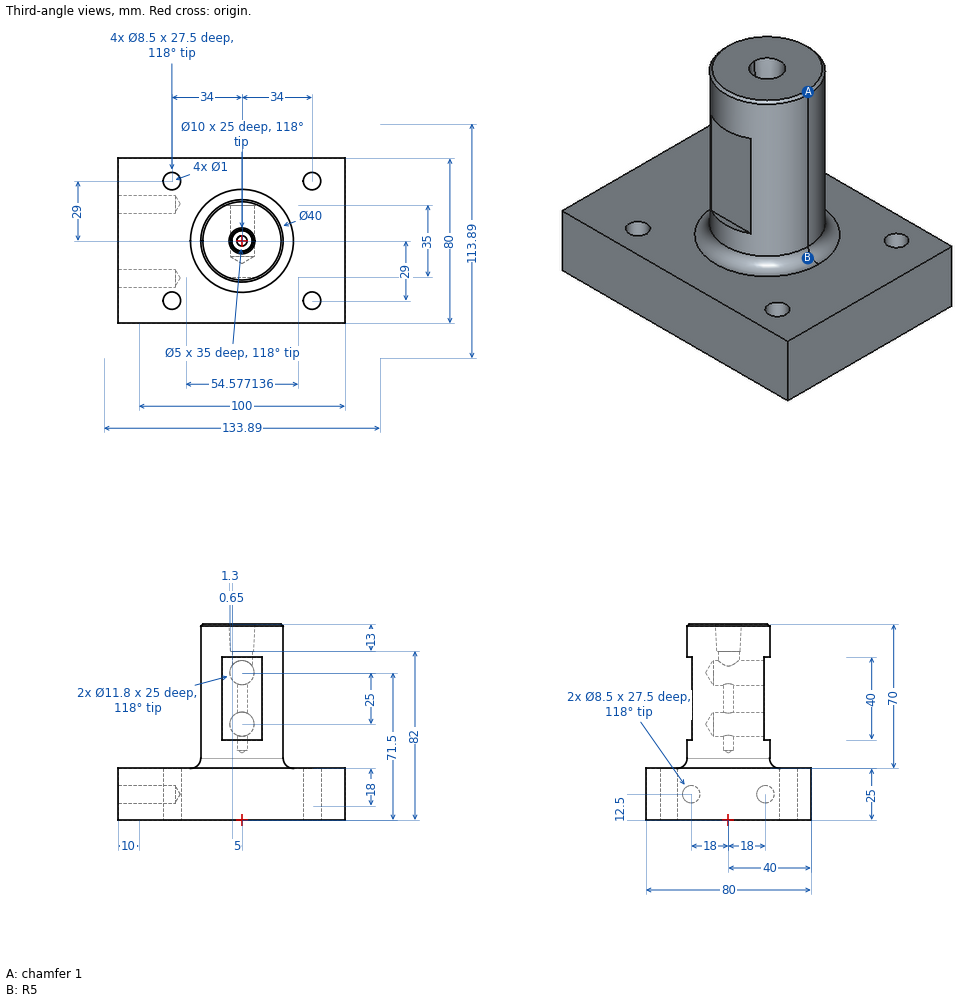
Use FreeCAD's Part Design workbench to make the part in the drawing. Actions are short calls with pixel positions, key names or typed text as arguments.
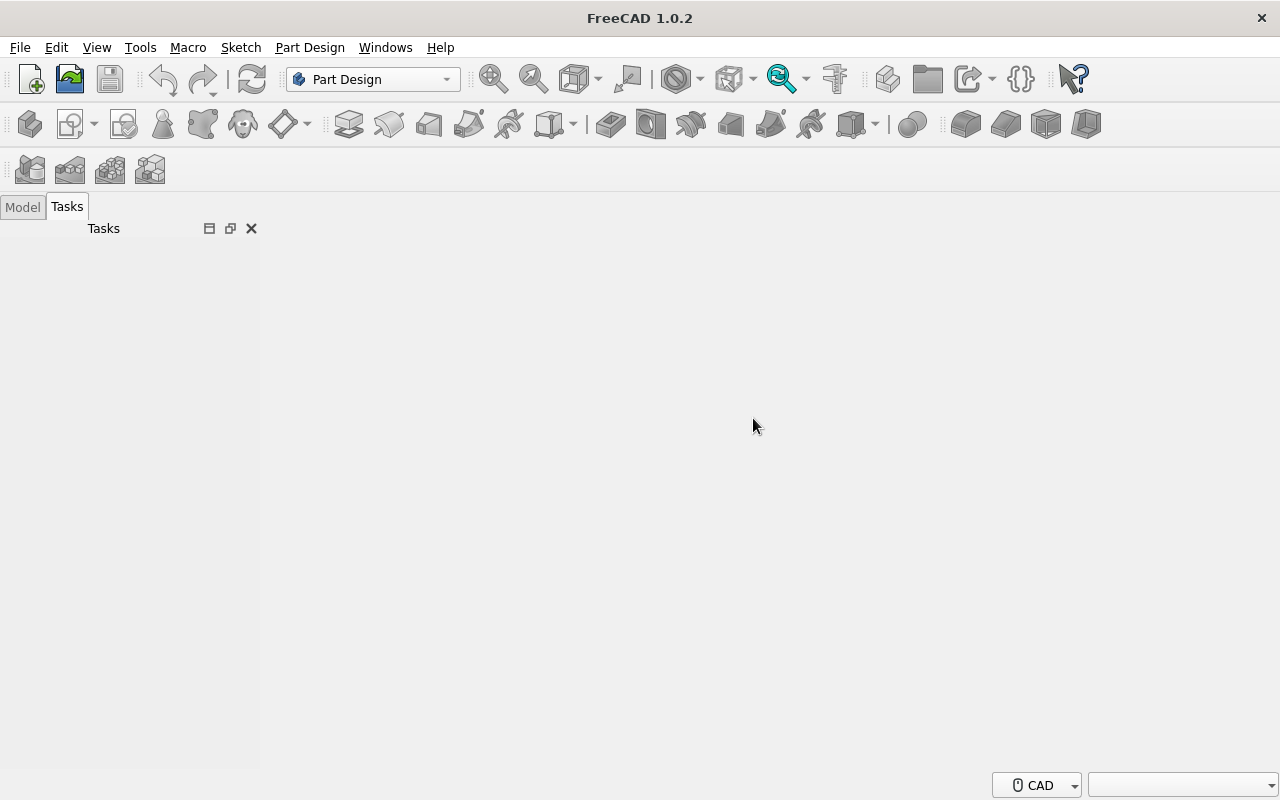
key(ctrl+n)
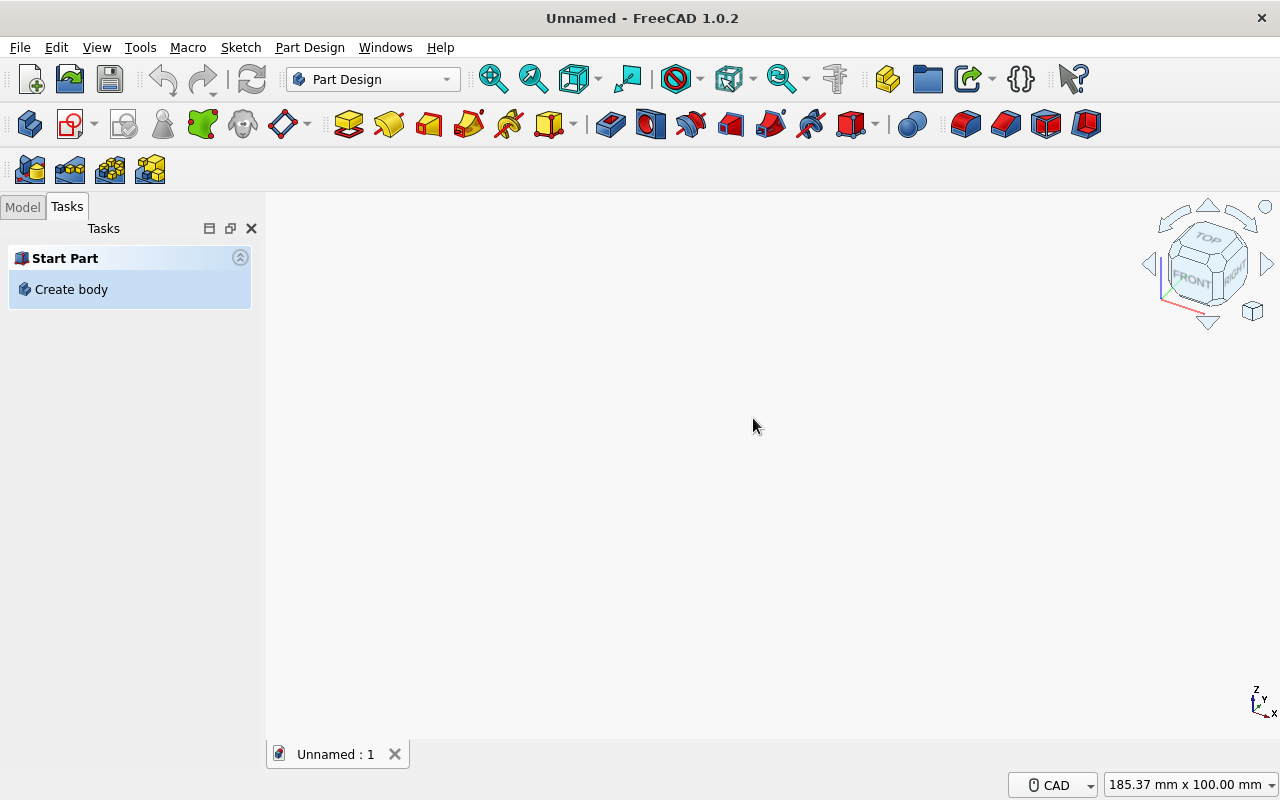
click(70, 124)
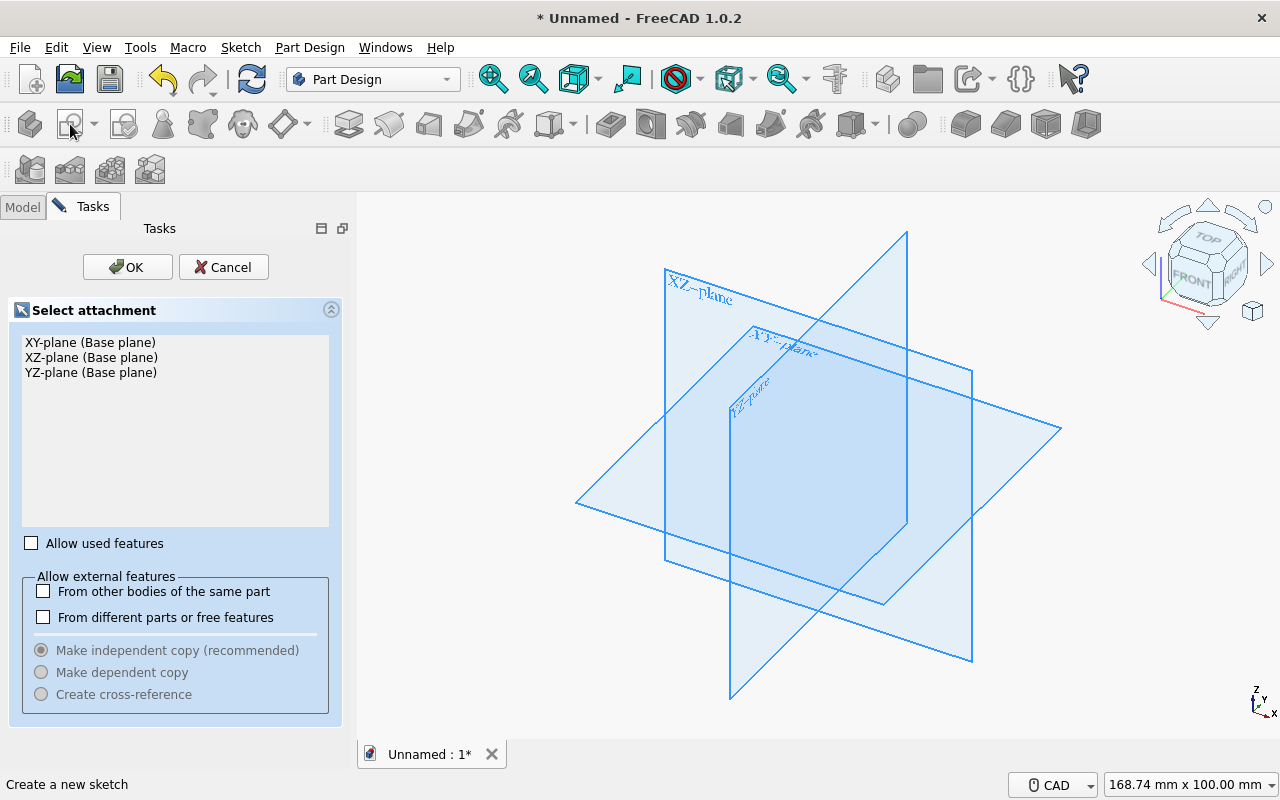
click(82, 342)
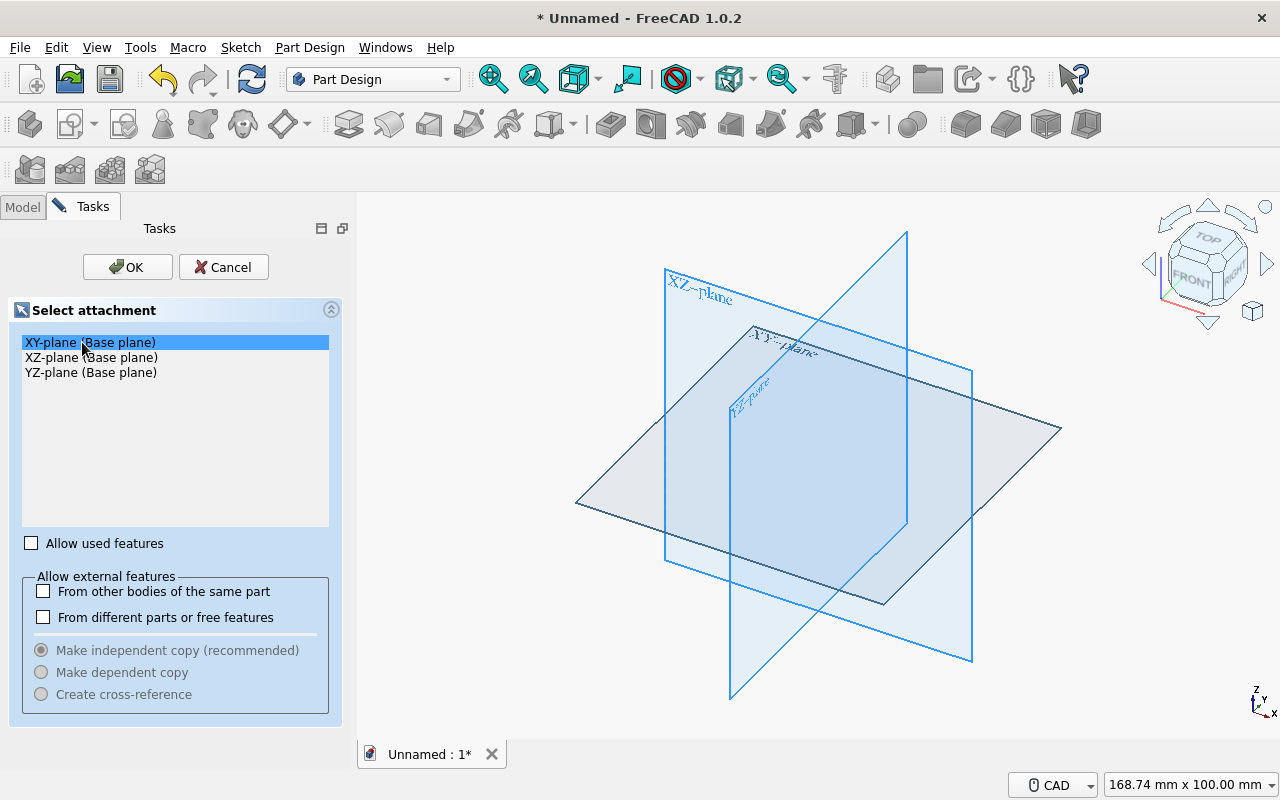
click(128, 267)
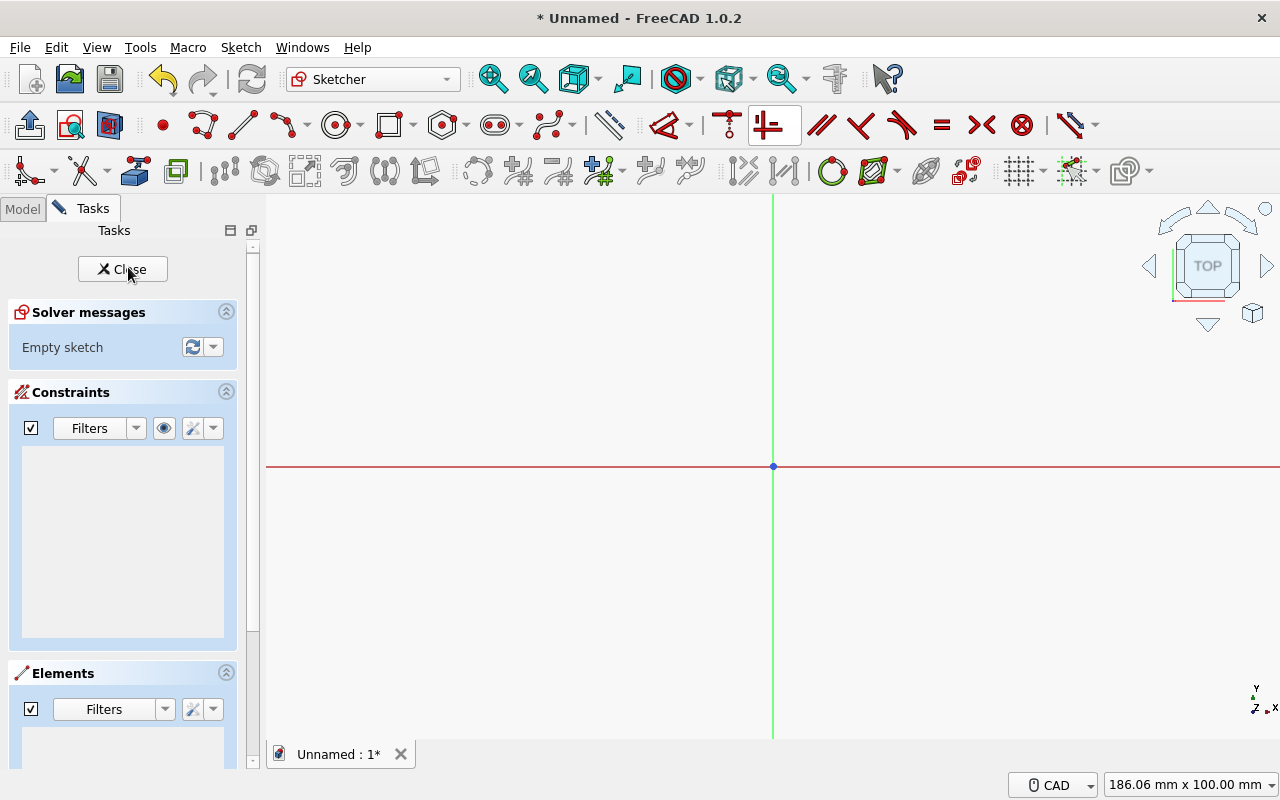
key(g)
key(v)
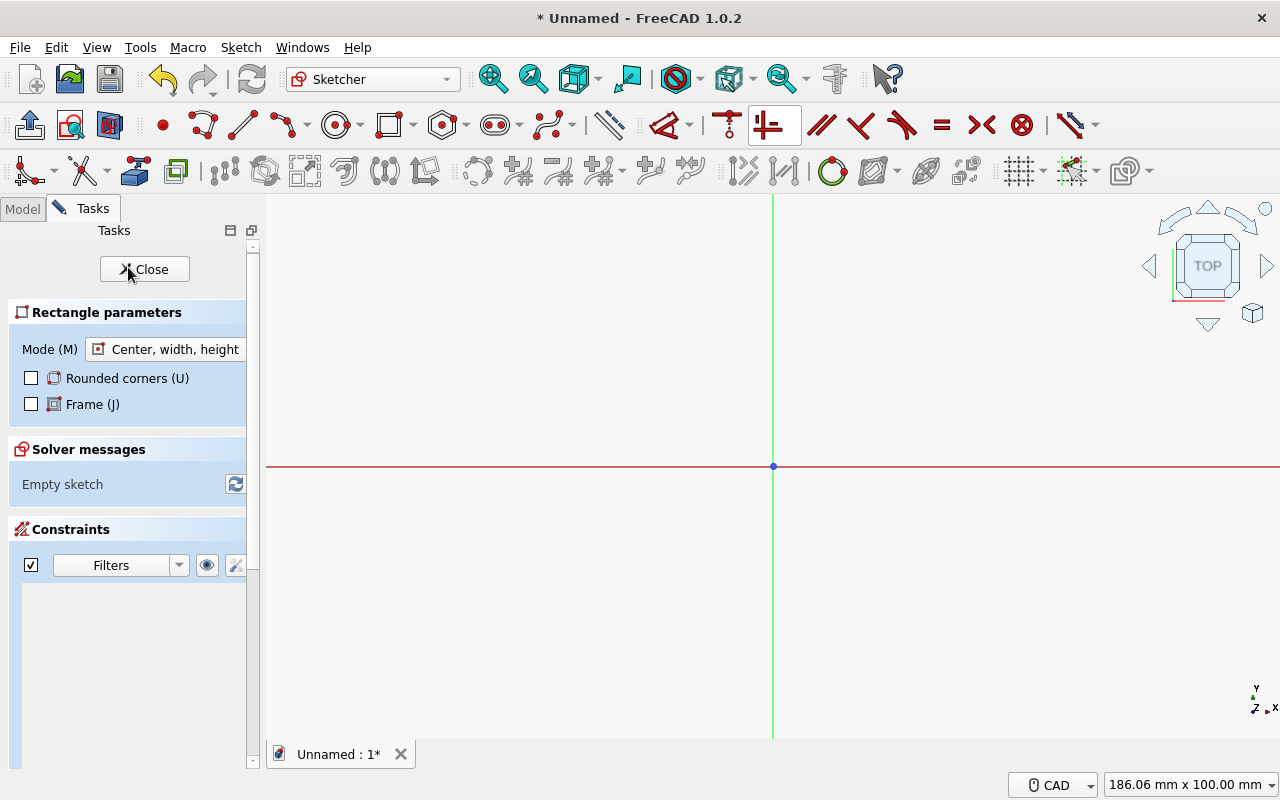
click(773, 466)
click(1046, 248)
key(Escape)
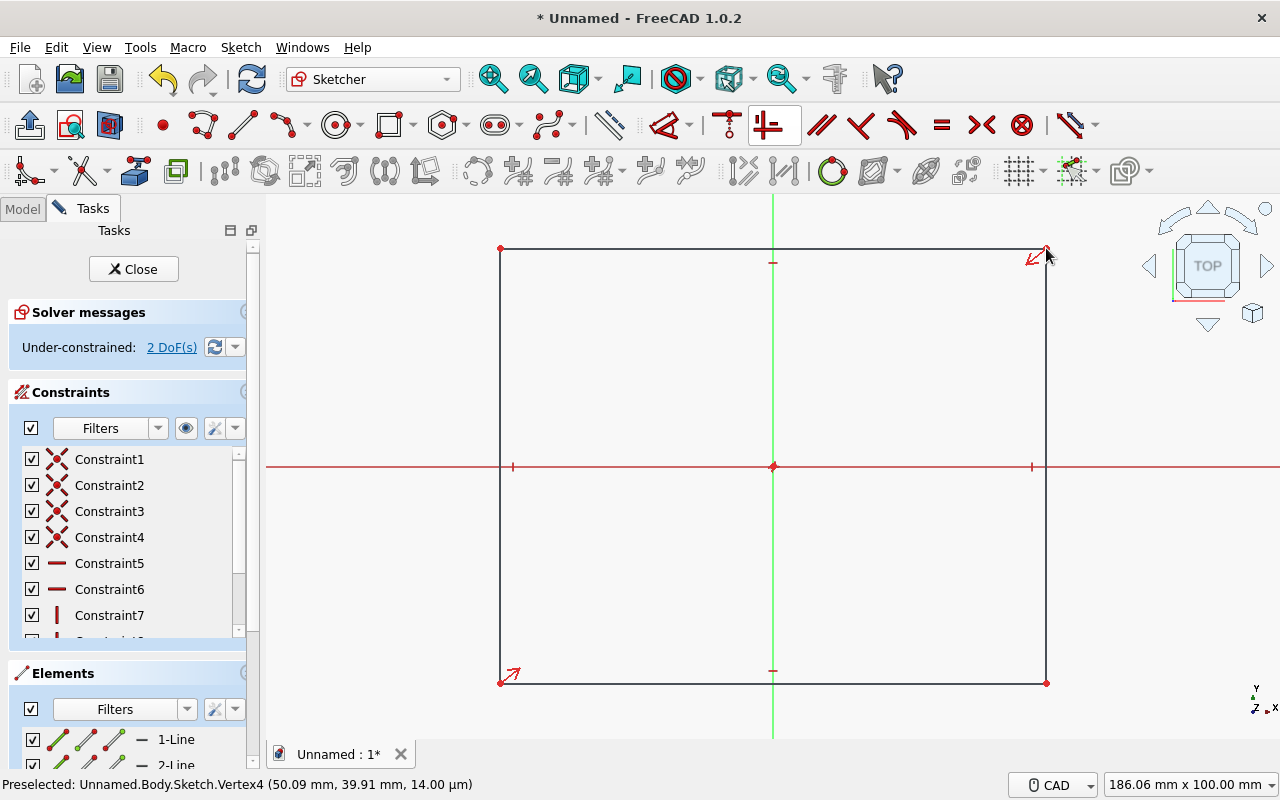
click(1046, 553)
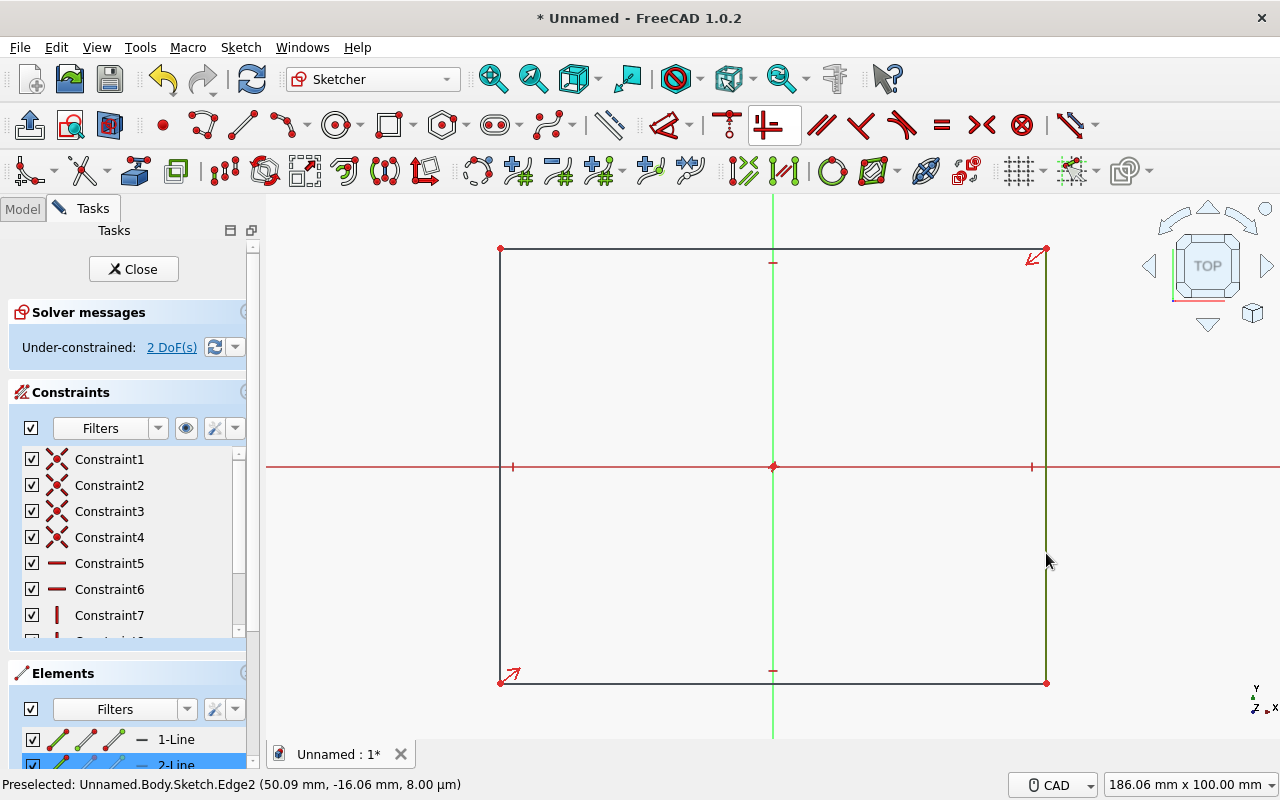
click(692, 126)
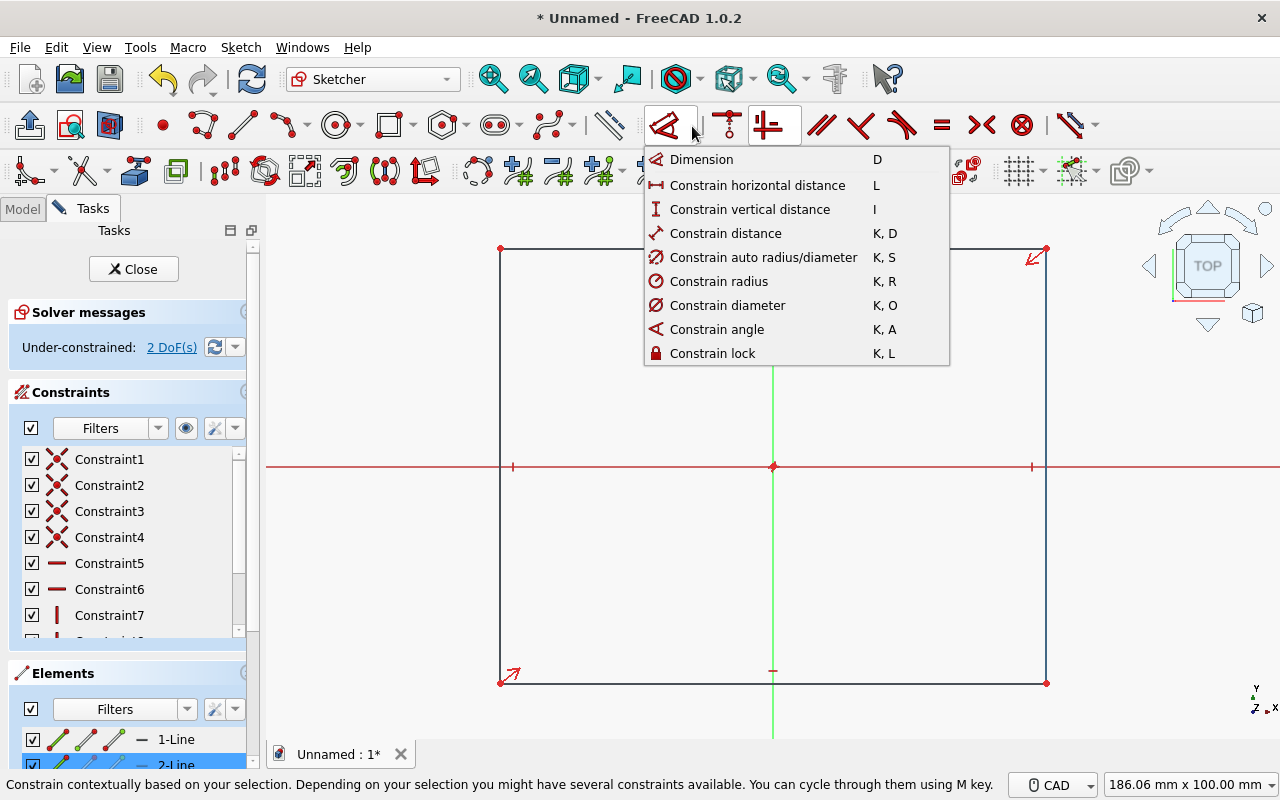
click(797, 209)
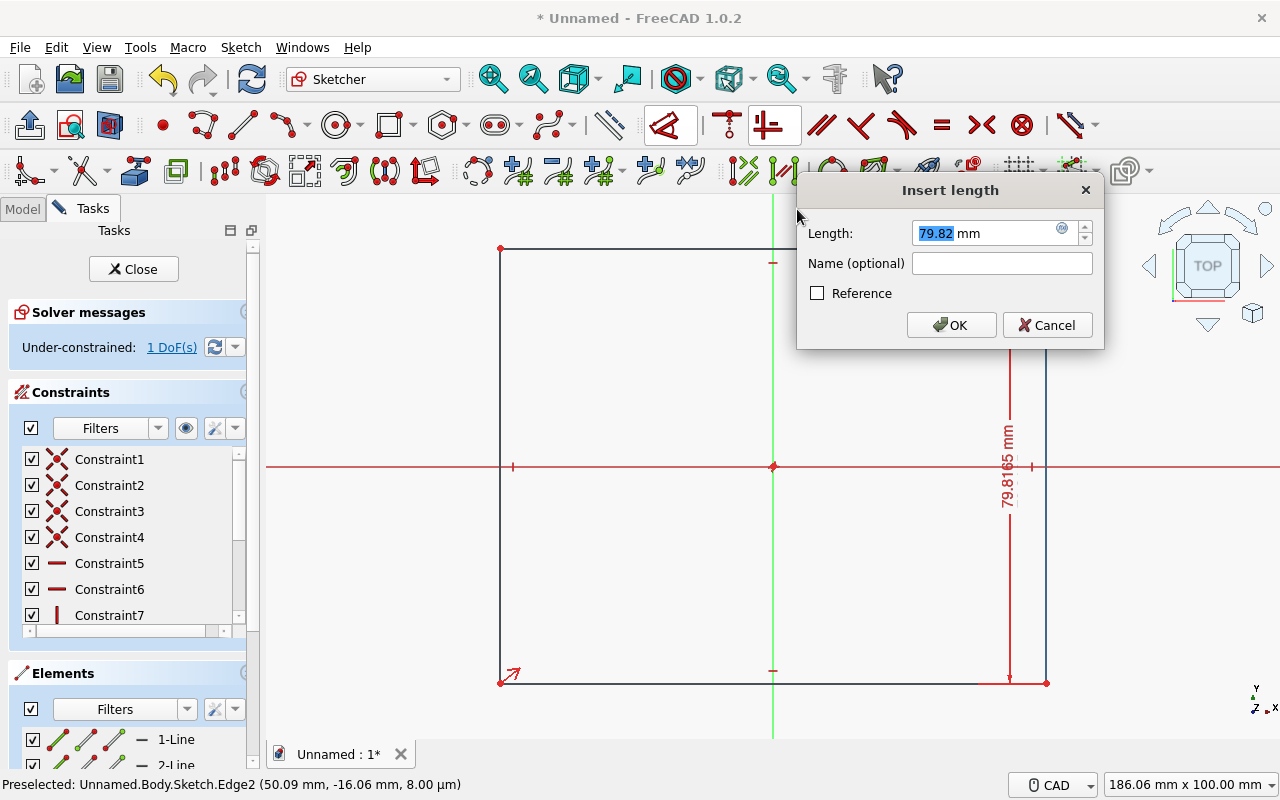
text(80)
key(Return)